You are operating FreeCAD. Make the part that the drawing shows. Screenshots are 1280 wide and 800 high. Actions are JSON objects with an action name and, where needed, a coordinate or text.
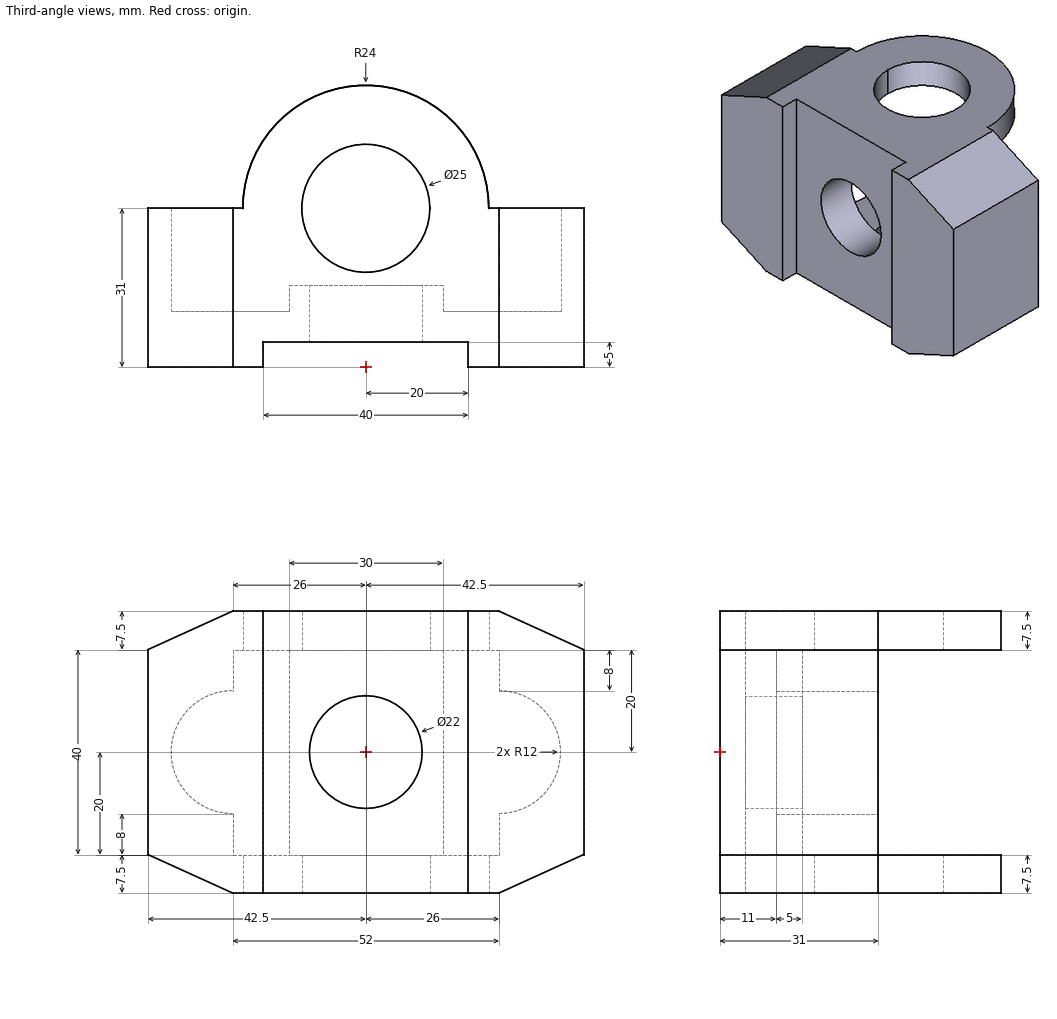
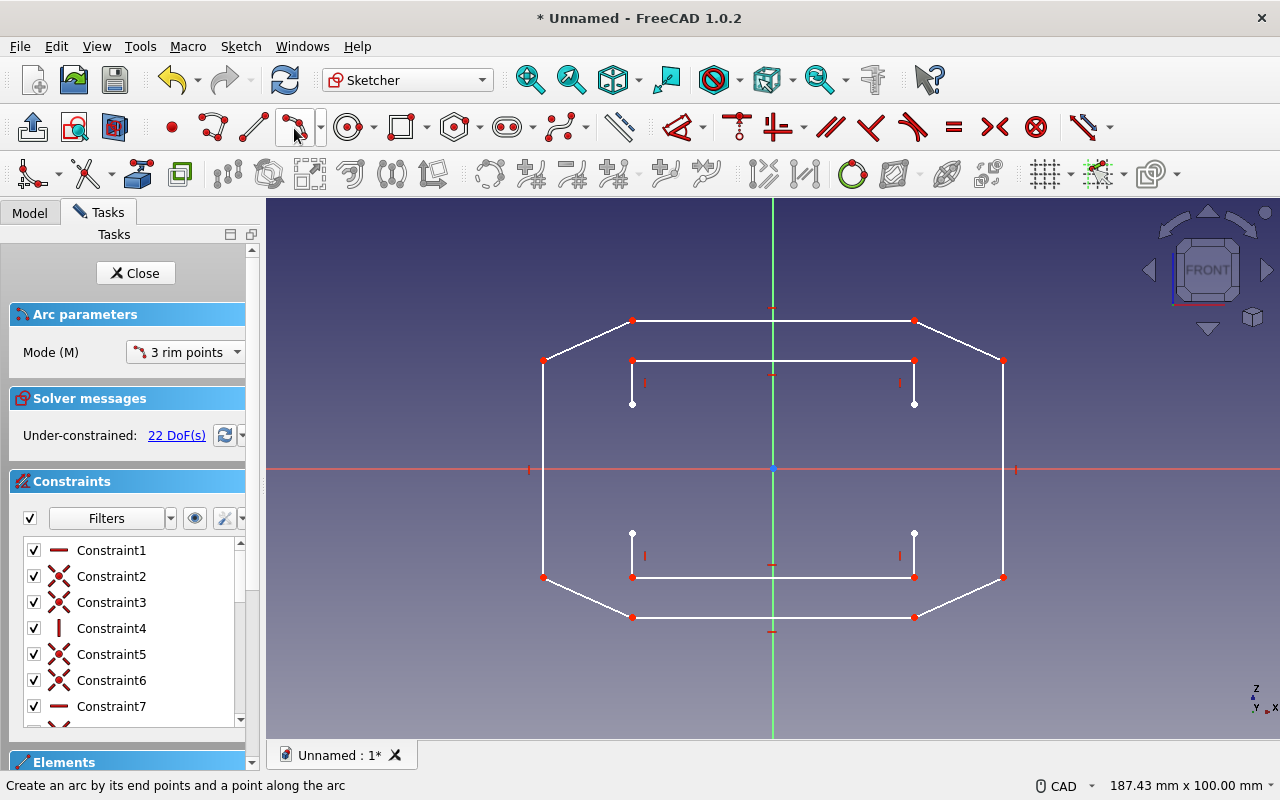
{"action": "left_click", "coordinate": [632, 405]}
{"action": "left_click", "coordinate": [632, 534]}
{"action": "left_click", "coordinate": [571, 448]}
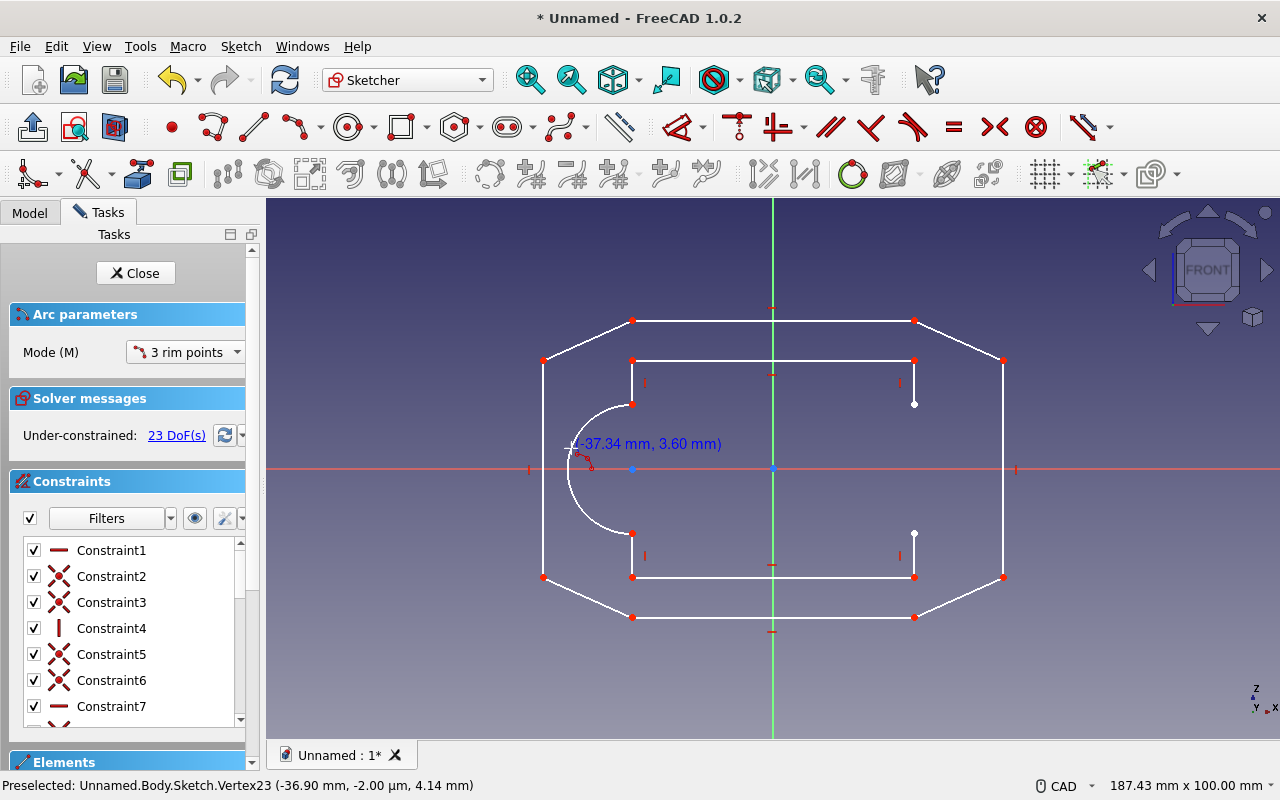
{"action": "left_click", "coordinate": [914, 534]}
{"action": "left_click", "coordinate": [914, 405]}
{"action": "left_click", "coordinate": [975, 489]}
{"action": "key", "text": "Escape"}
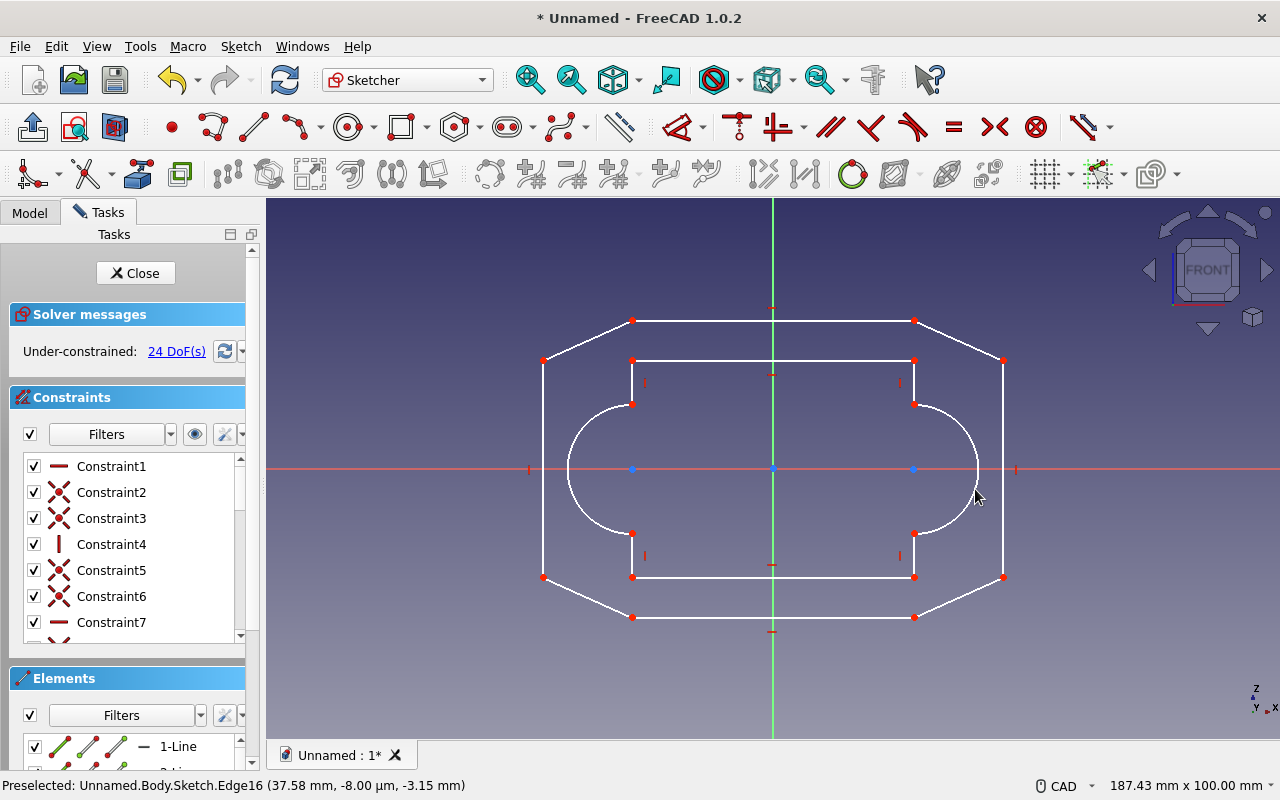
{"action": "left_click", "coordinate": [580, 432]}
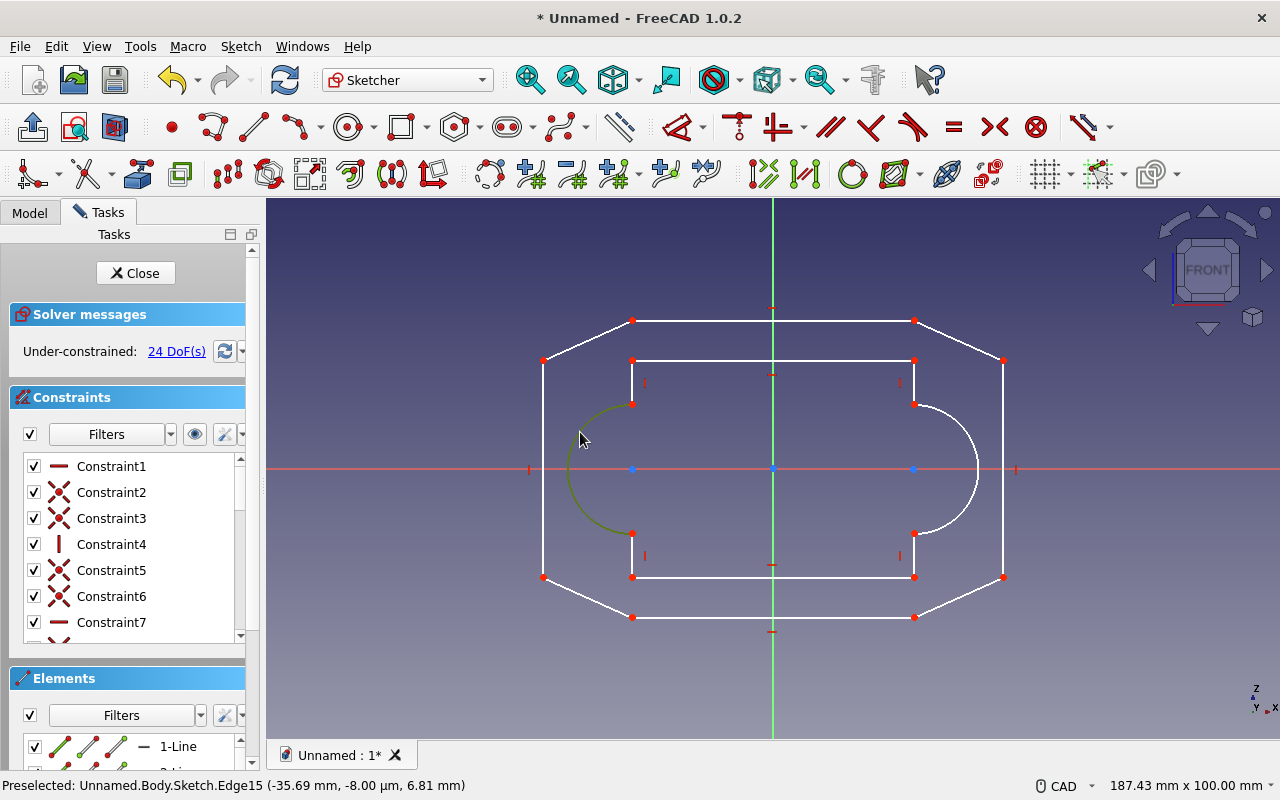
{"action": "left_click", "coordinate": [966, 507]}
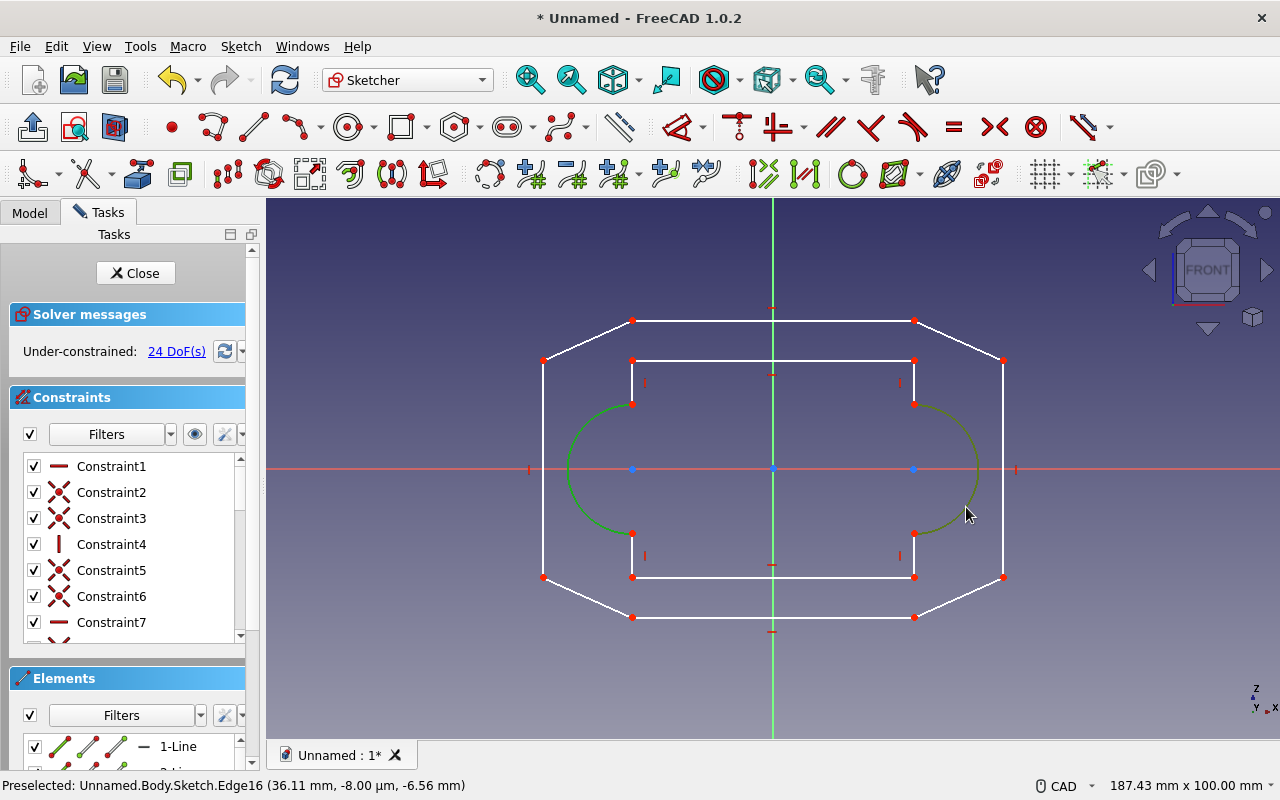
{"action": "left_click", "coordinate": [954, 128]}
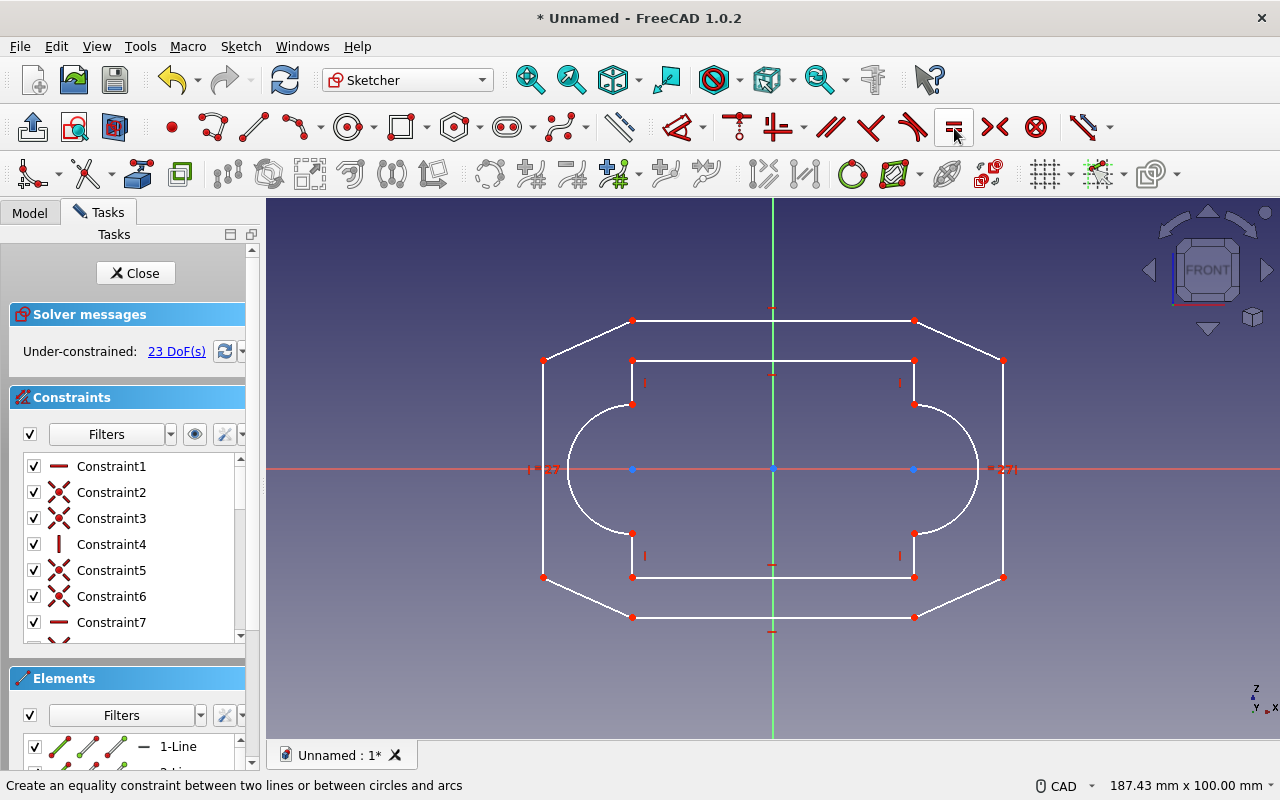
{"action": "left_click", "coordinate": [632, 469]}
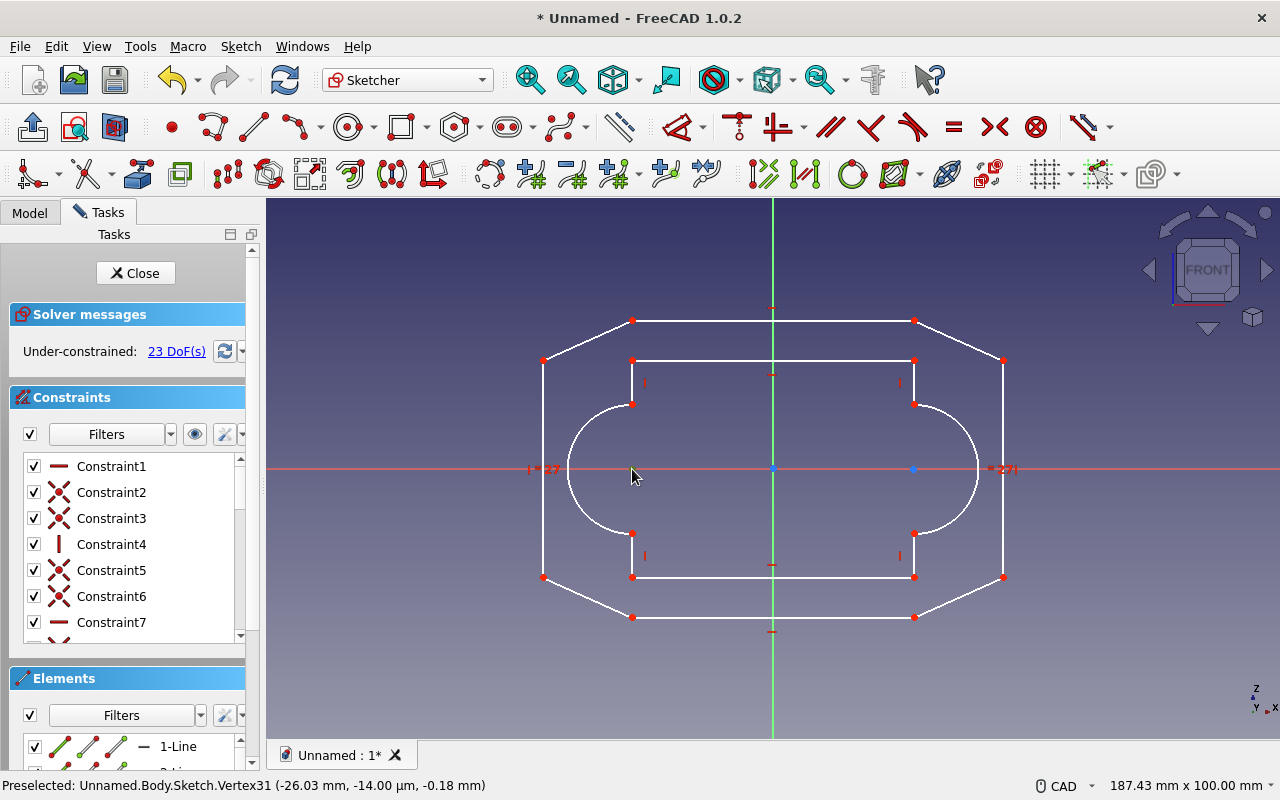
{"action": "left_click", "coordinate": [353, 468]}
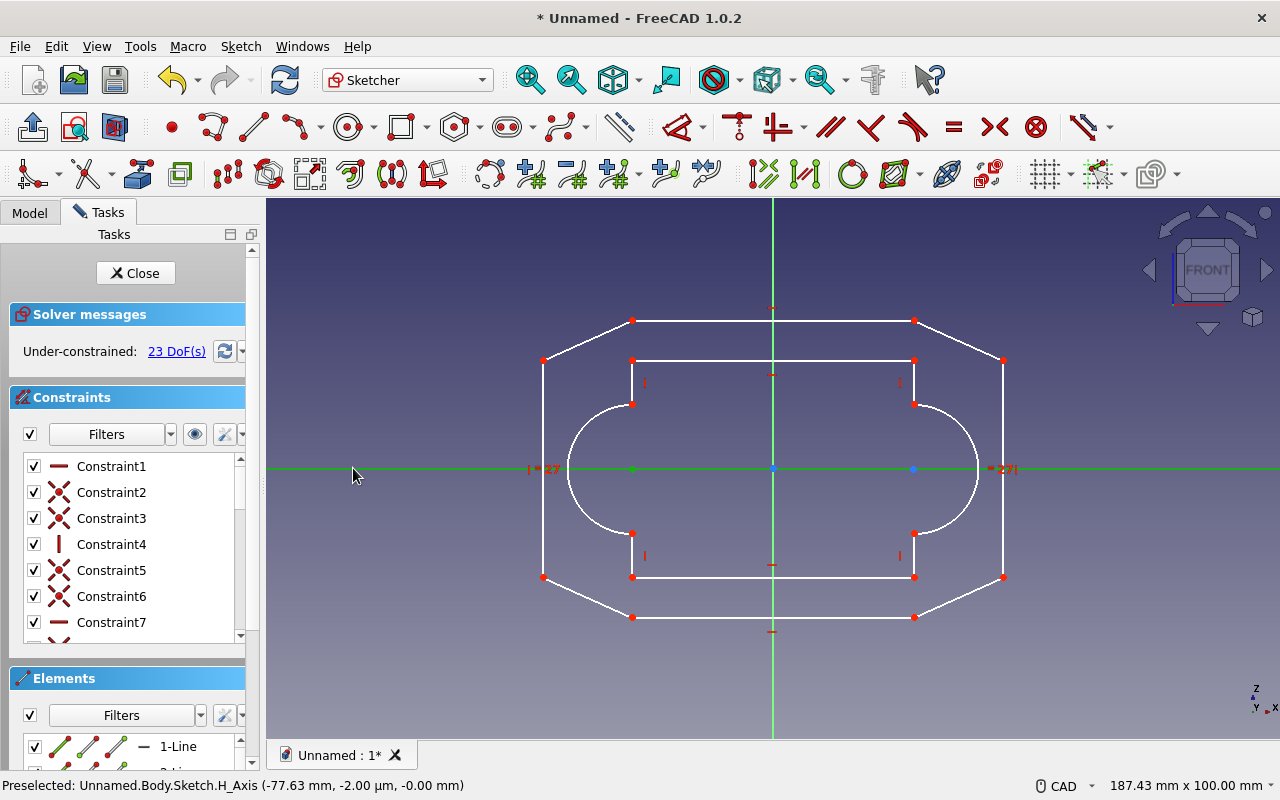
{"action": "left_click", "coordinate": [737, 128]}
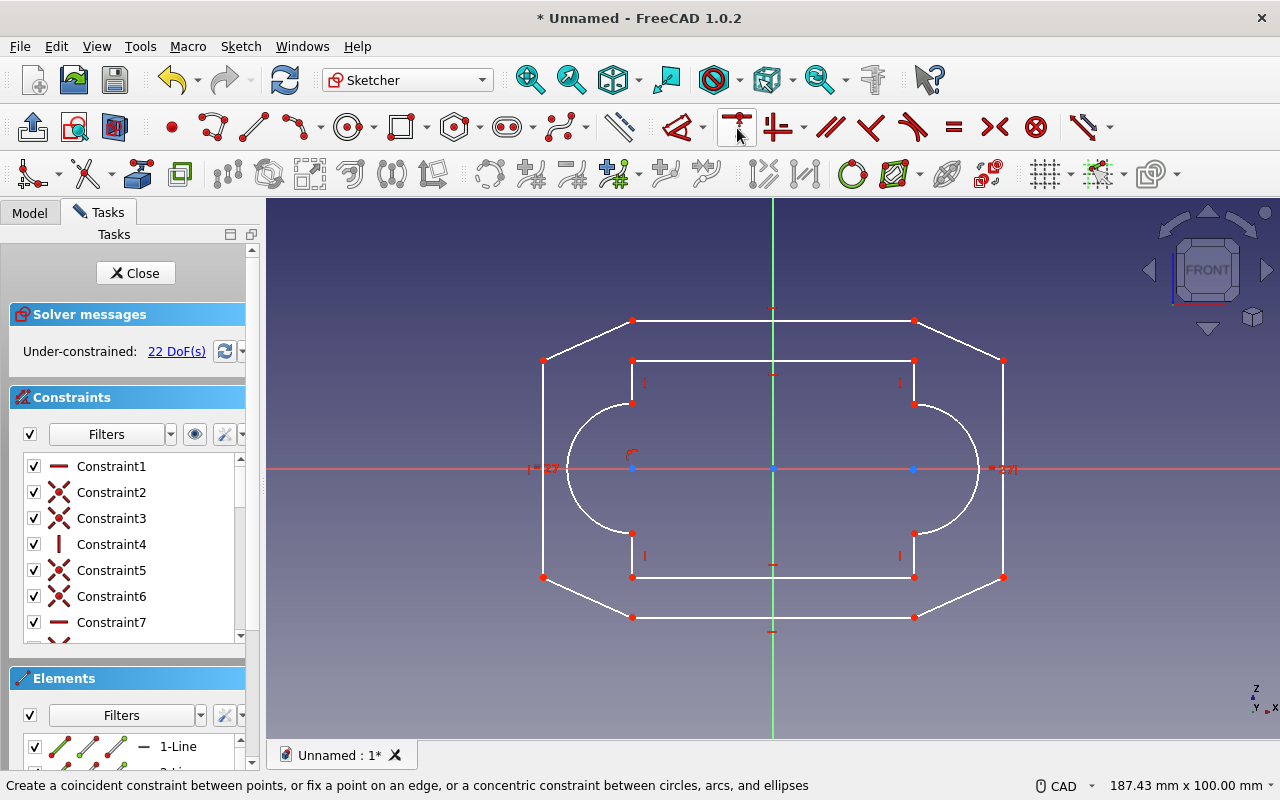
{"action": "left_click", "coordinate": [914, 469]}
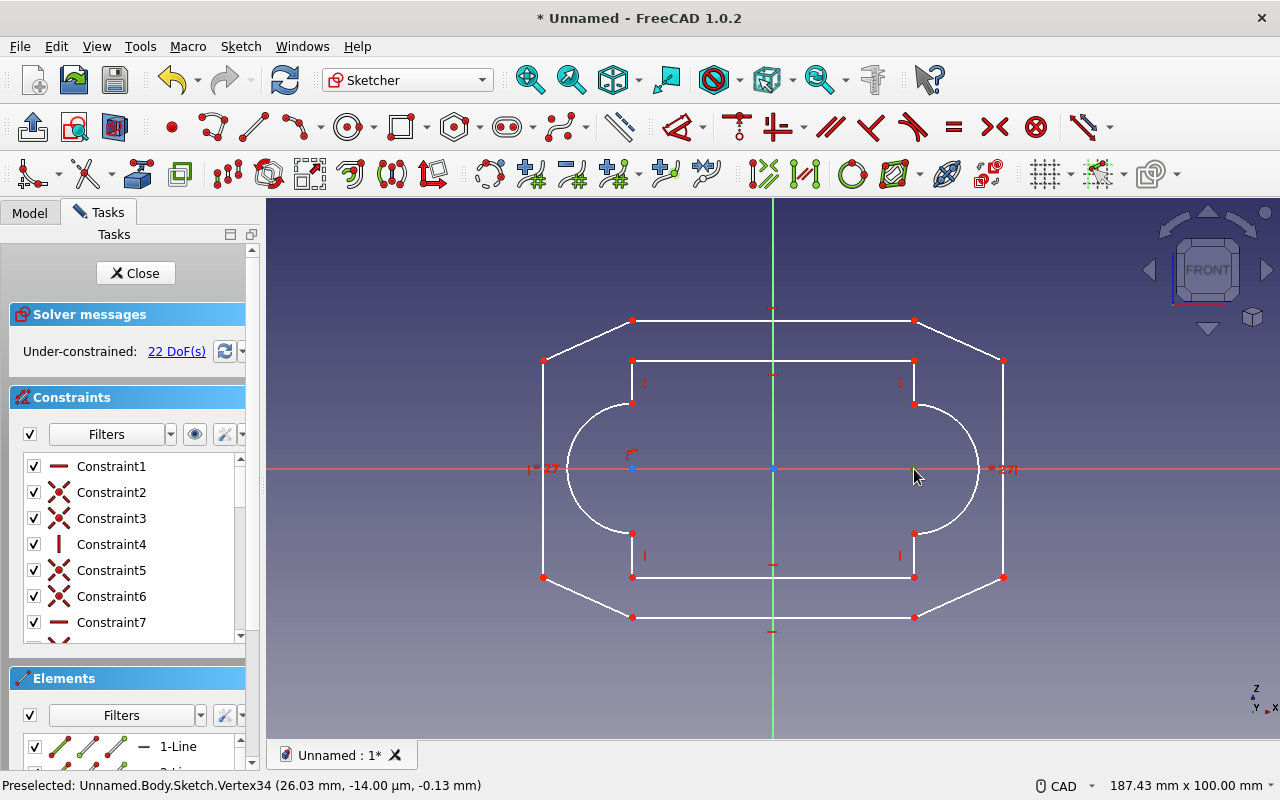
{"action": "left_click", "coordinate": [353, 468]}